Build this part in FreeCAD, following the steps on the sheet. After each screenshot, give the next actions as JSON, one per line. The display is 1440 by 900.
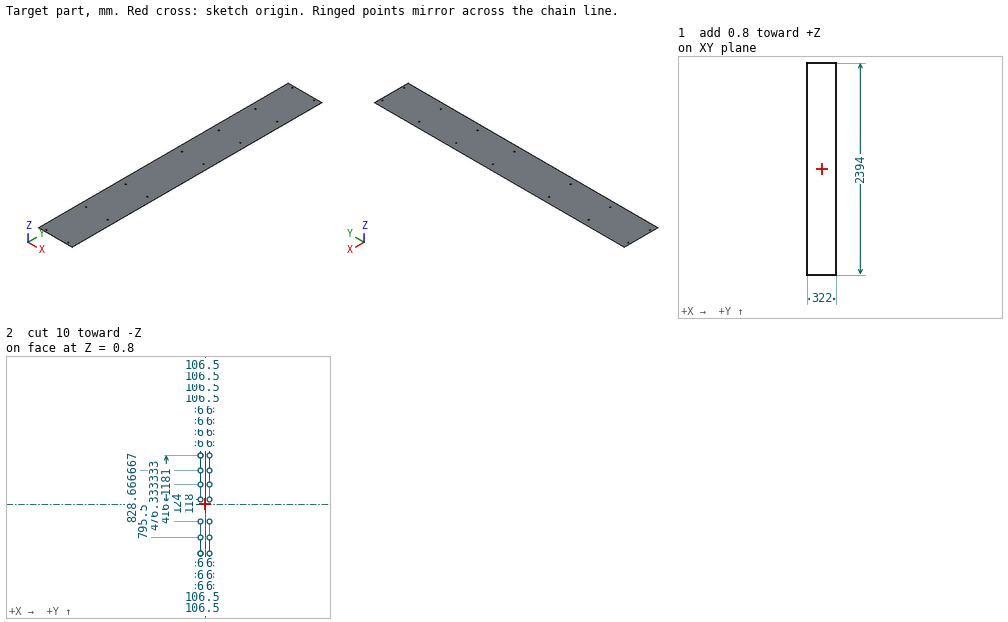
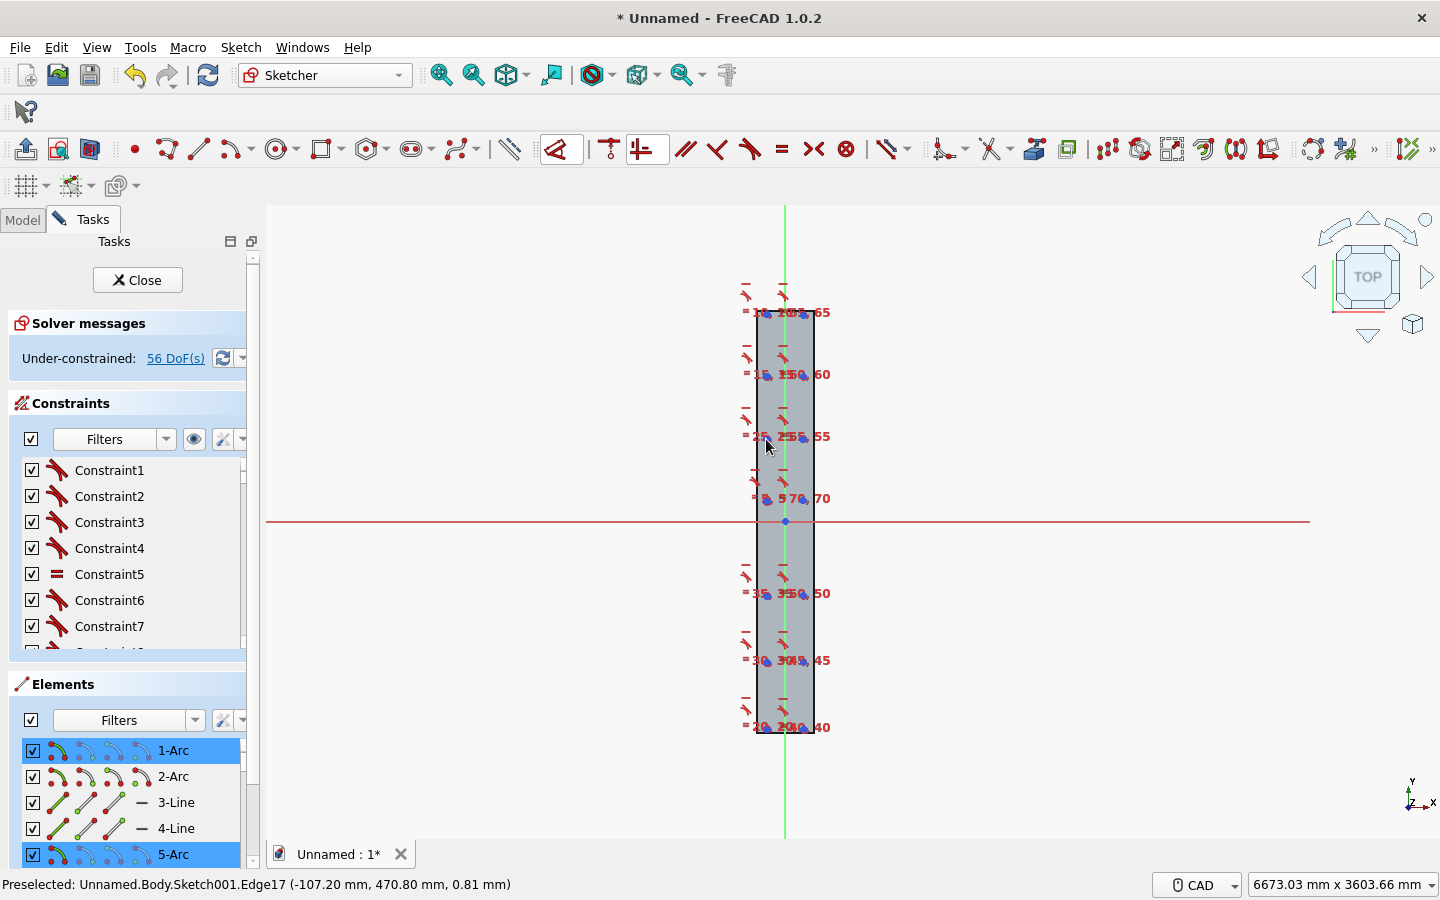
{"action": "scroll", "coordinate": [766, 663], "scroll_direction": "up", "scroll_amount": 14}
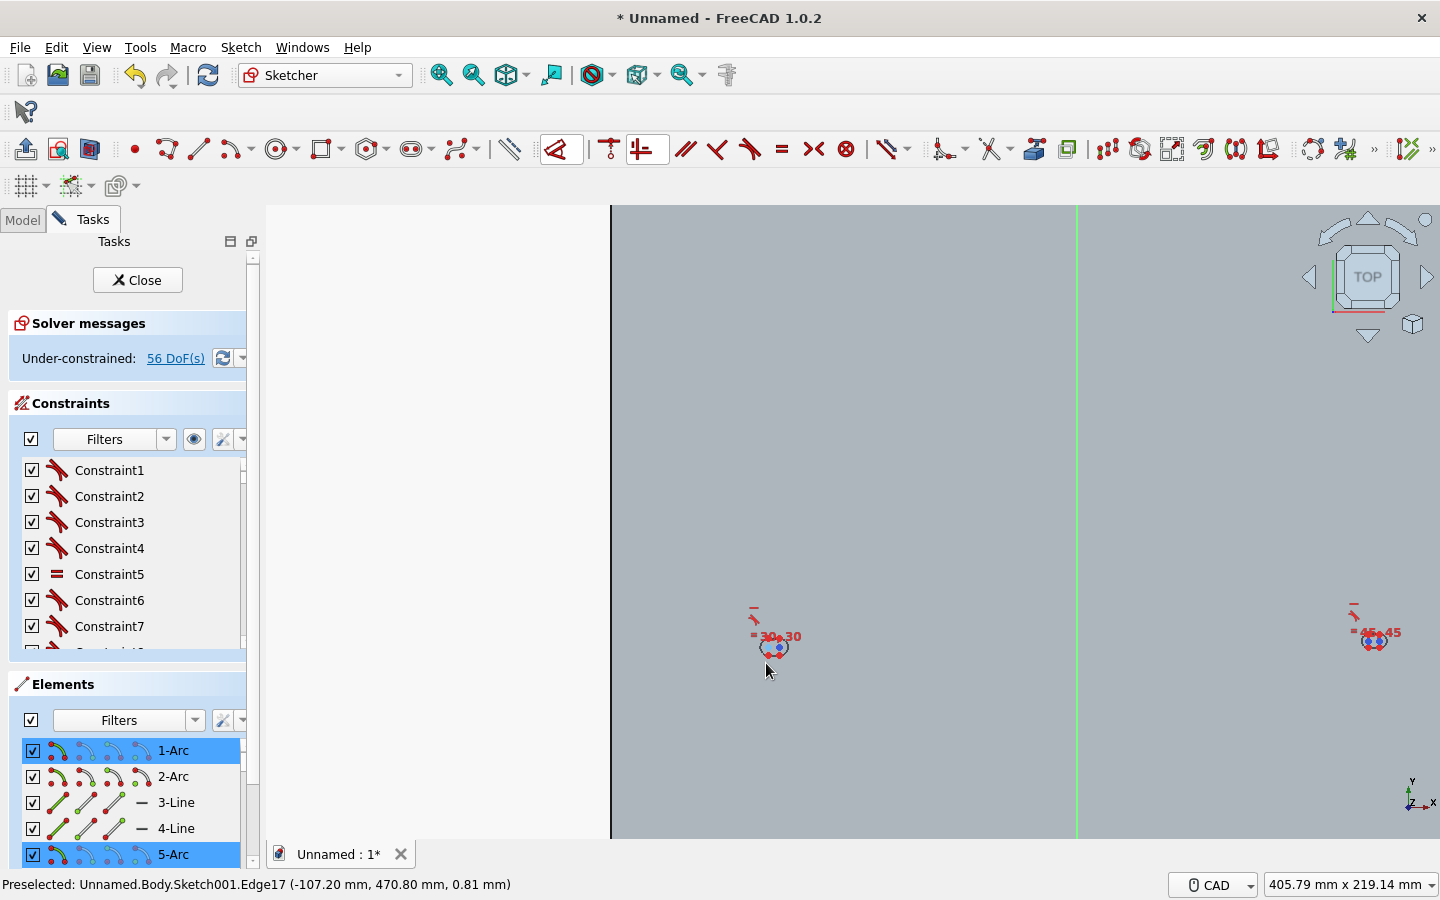
{"action": "left_click", "coordinate": [760, 647]}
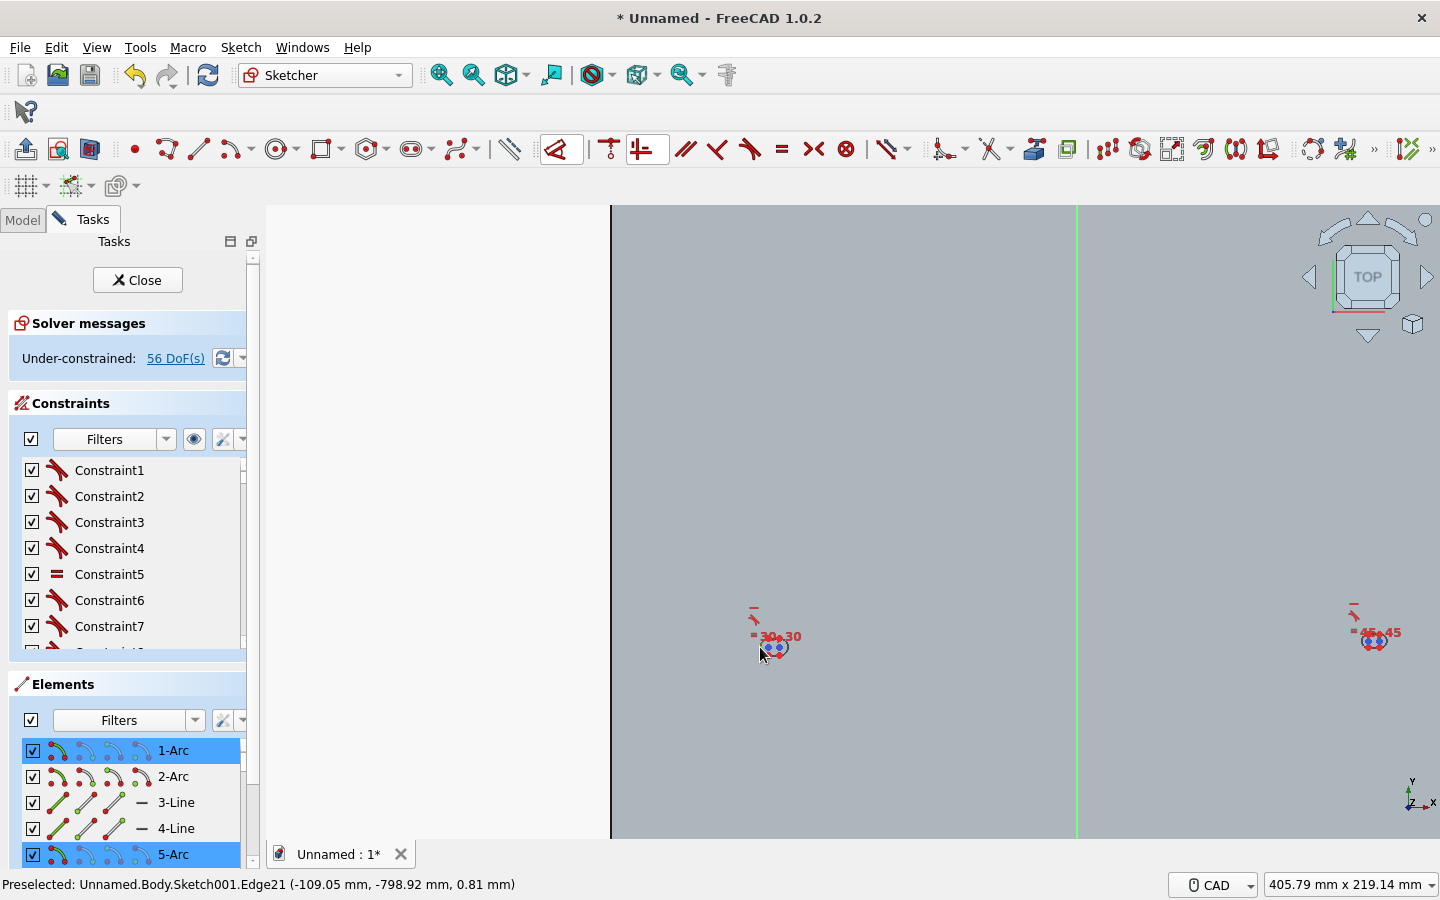
{"action": "scroll", "coordinate": [766, 664], "scroll_direction": "down", "scroll_amount": 14}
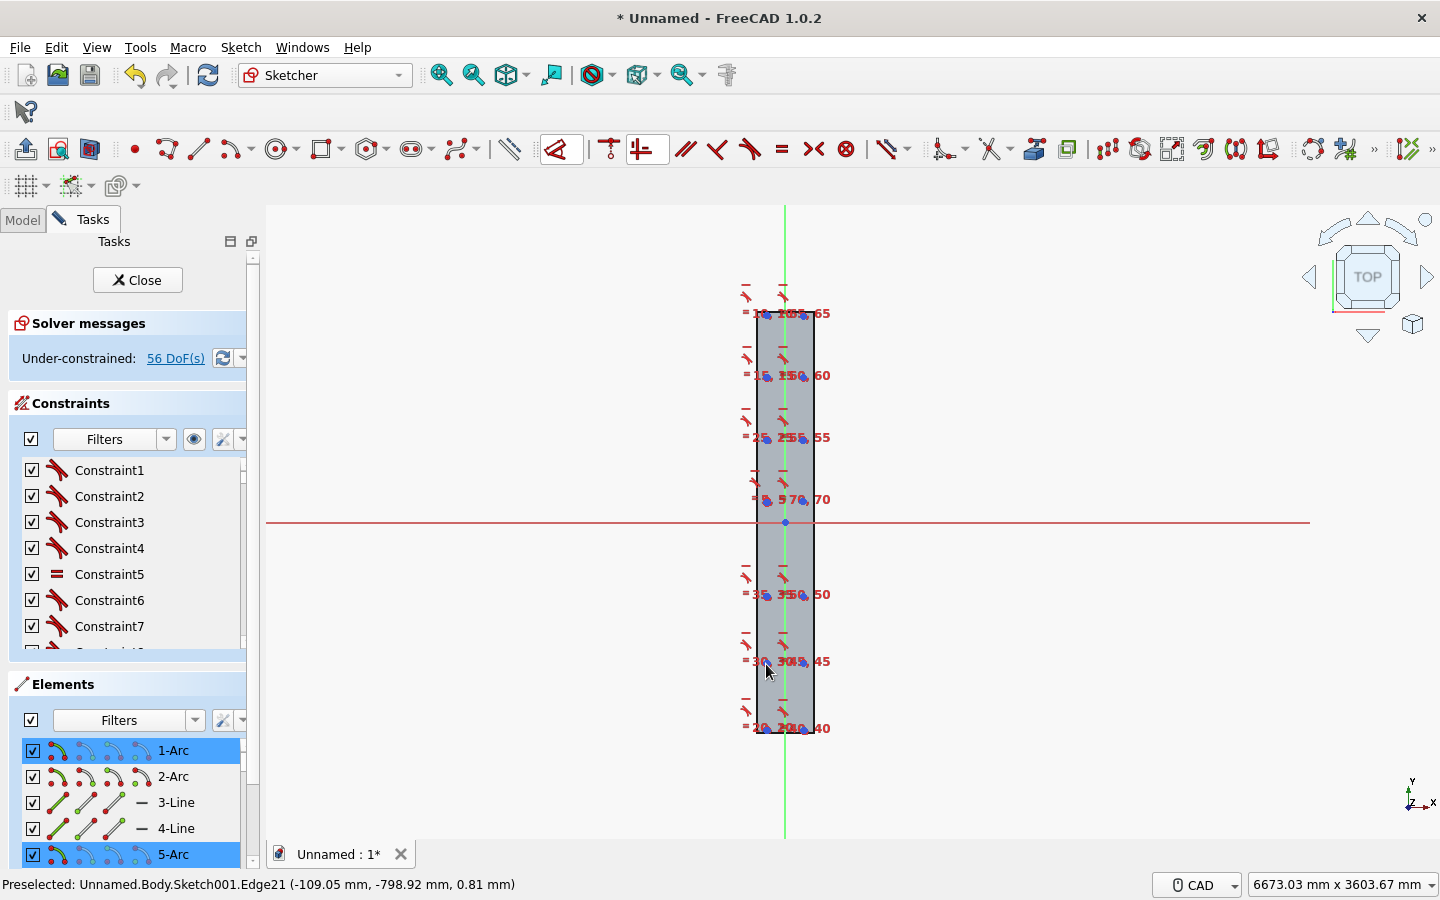
{"action": "scroll", "coordinate": [766, 597], "scroll_direction": "up", "scroll_amount": 14}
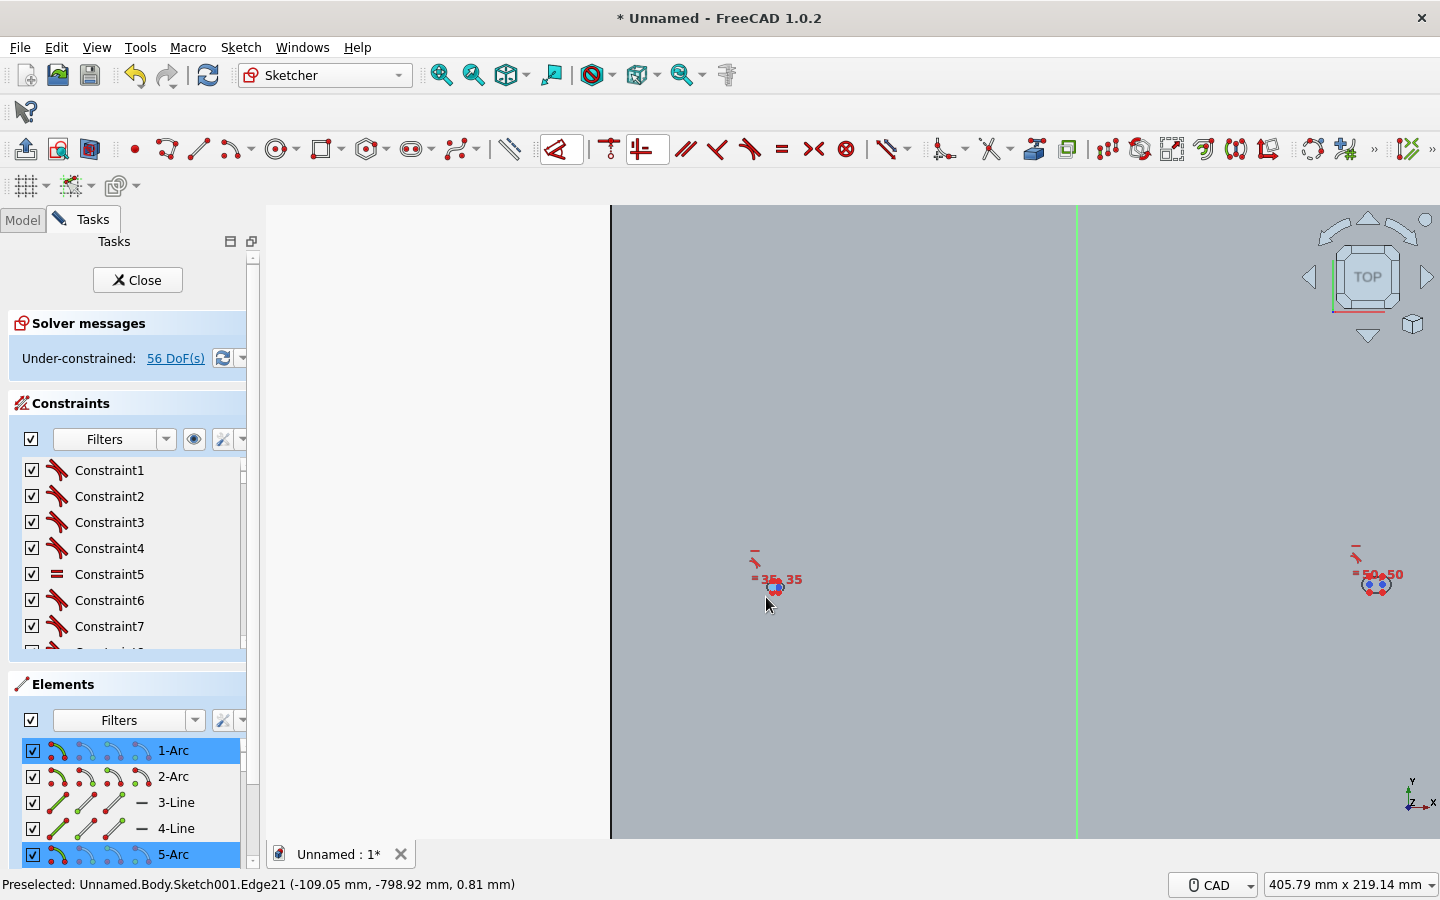
{"action": "left_click", "coordinate": [767, 587]}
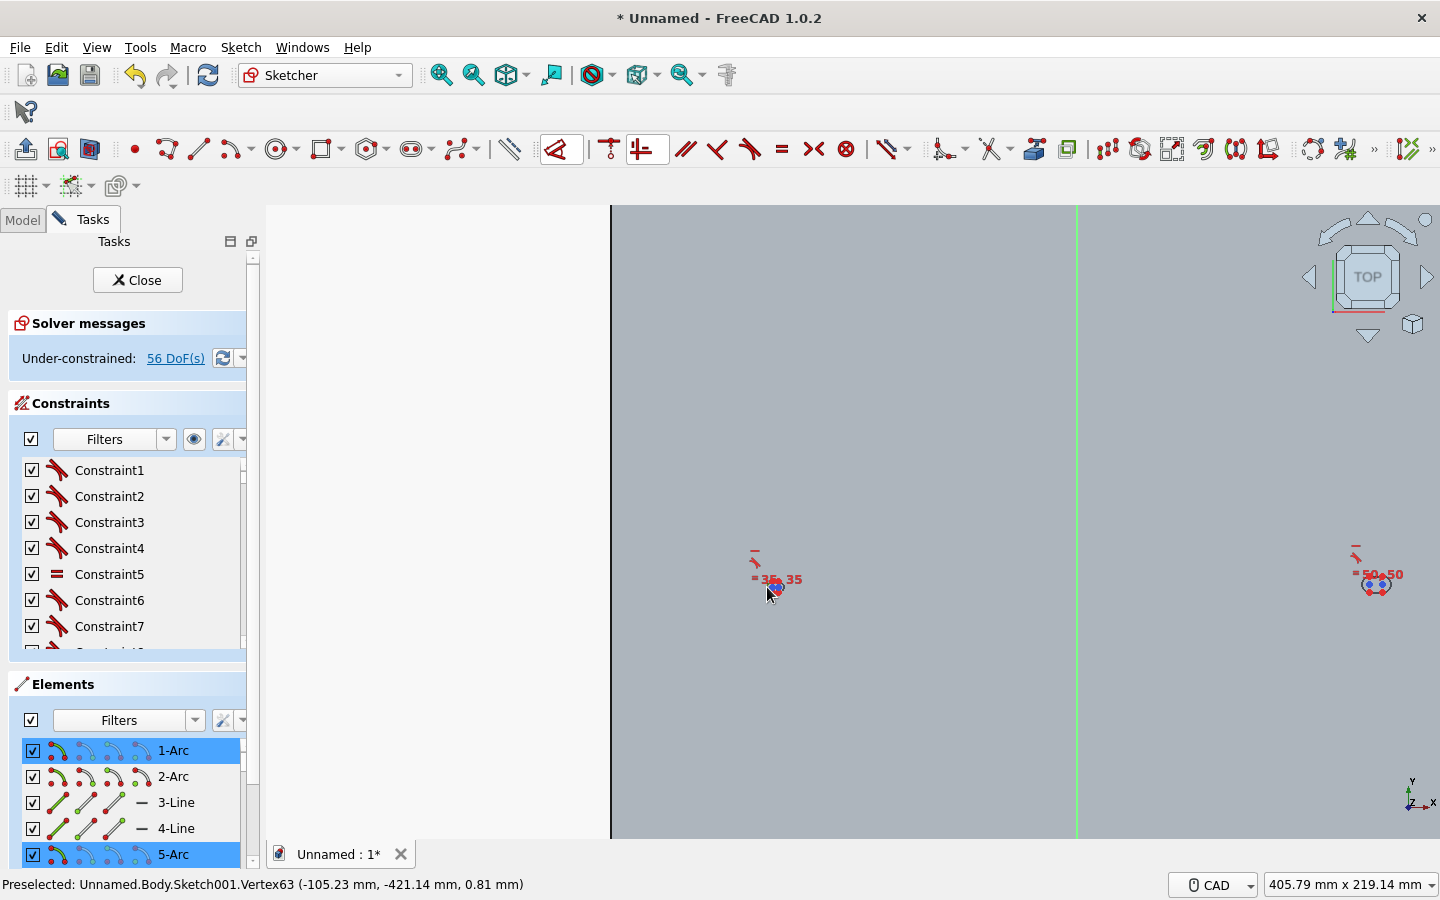
{"action": "scroll", "coordinate": [766, 597], "scroll_direction": "down", "scroll_amount": 14}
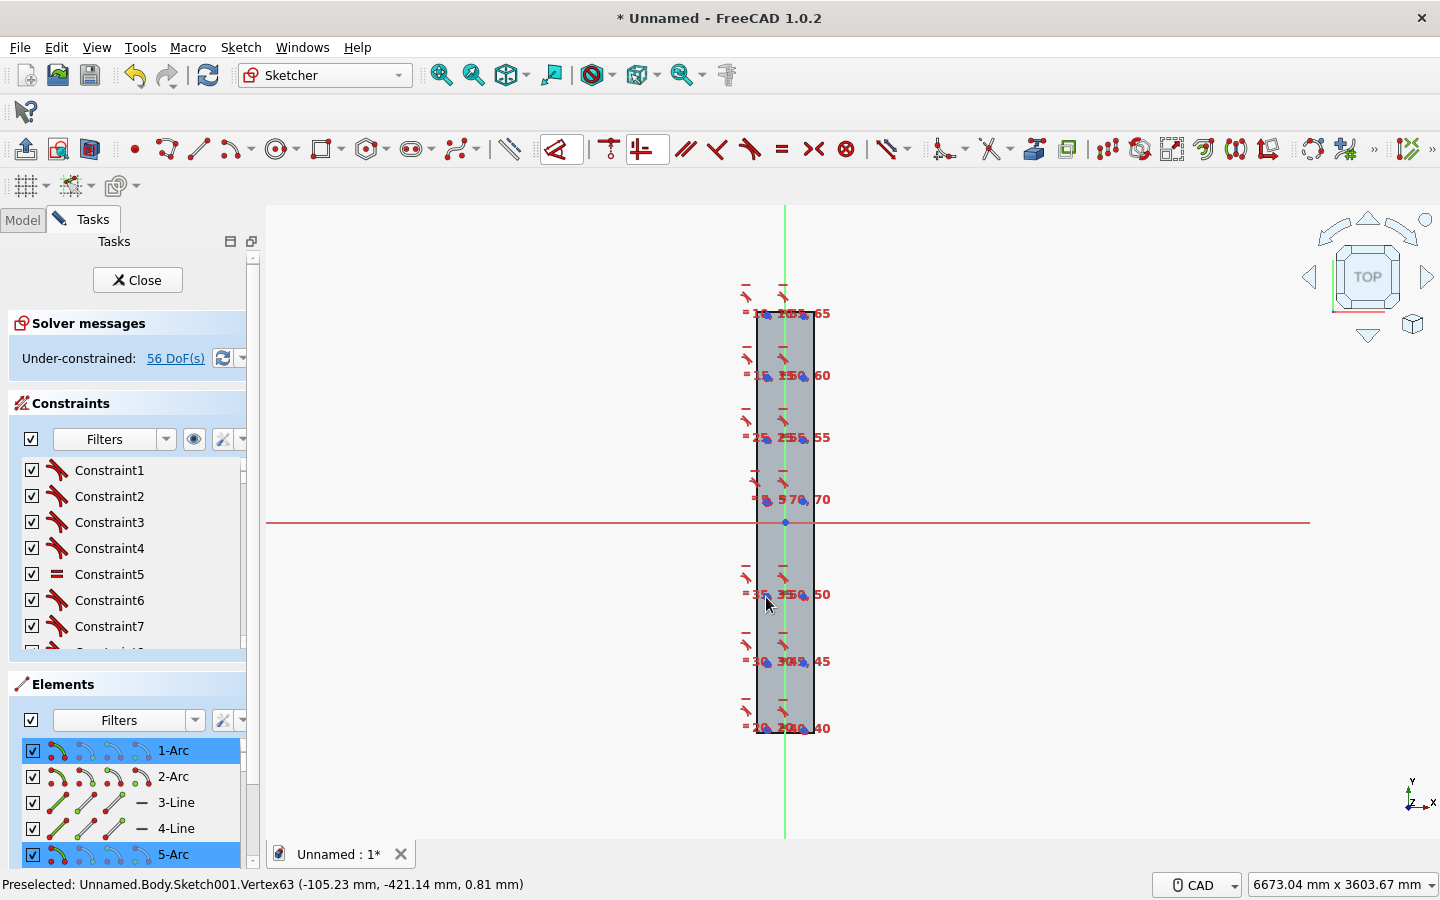
{"action": "scroll", "coordinate": [803, 730], "scroll_direction": "up", "scroll_amount": 14}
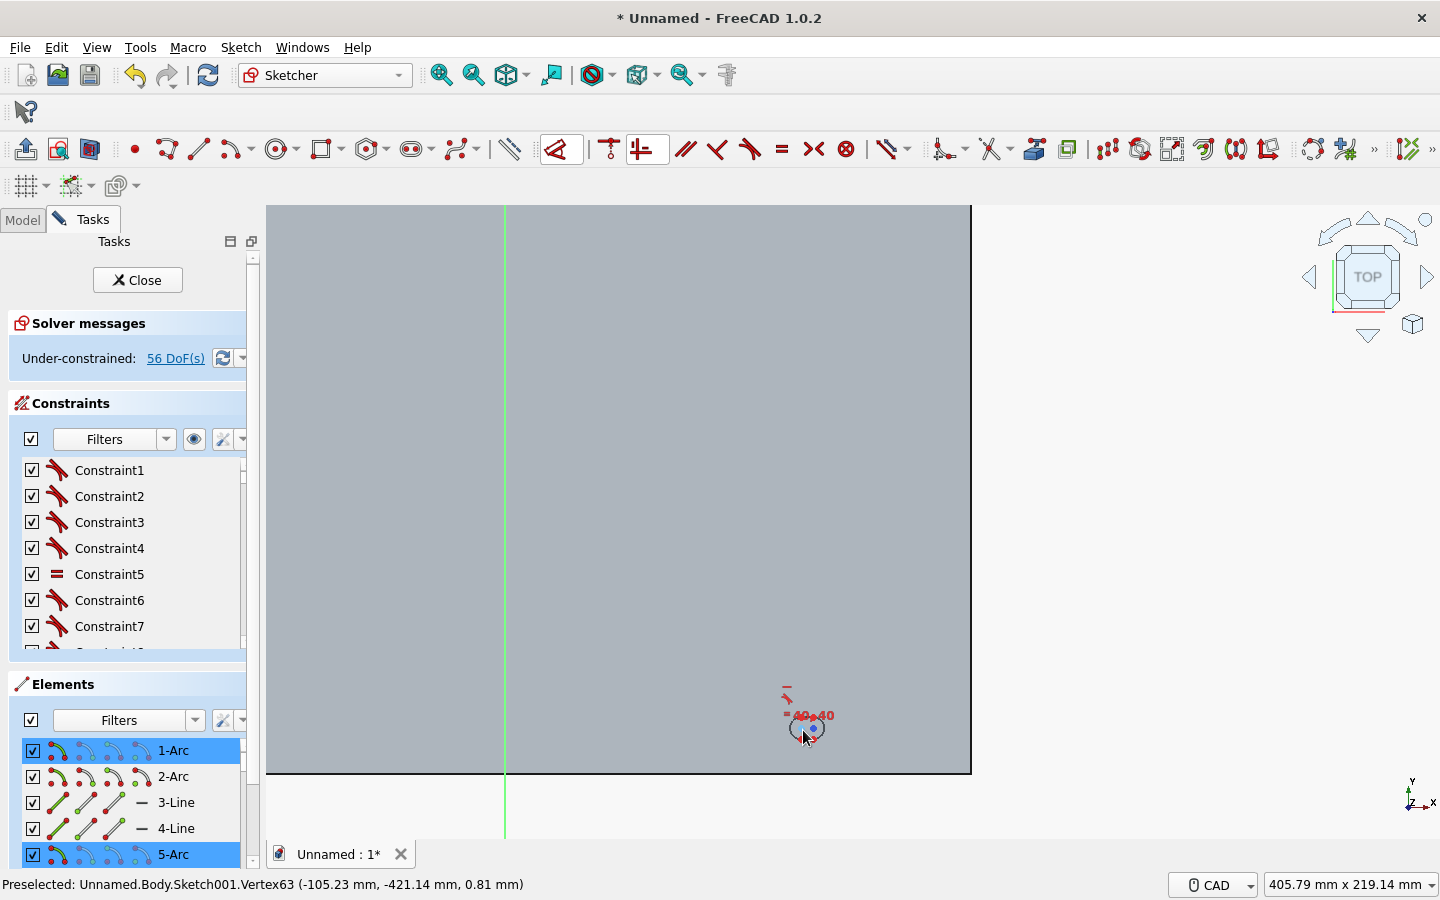
{"action": "left_click", "coordinate": [792, 722]}